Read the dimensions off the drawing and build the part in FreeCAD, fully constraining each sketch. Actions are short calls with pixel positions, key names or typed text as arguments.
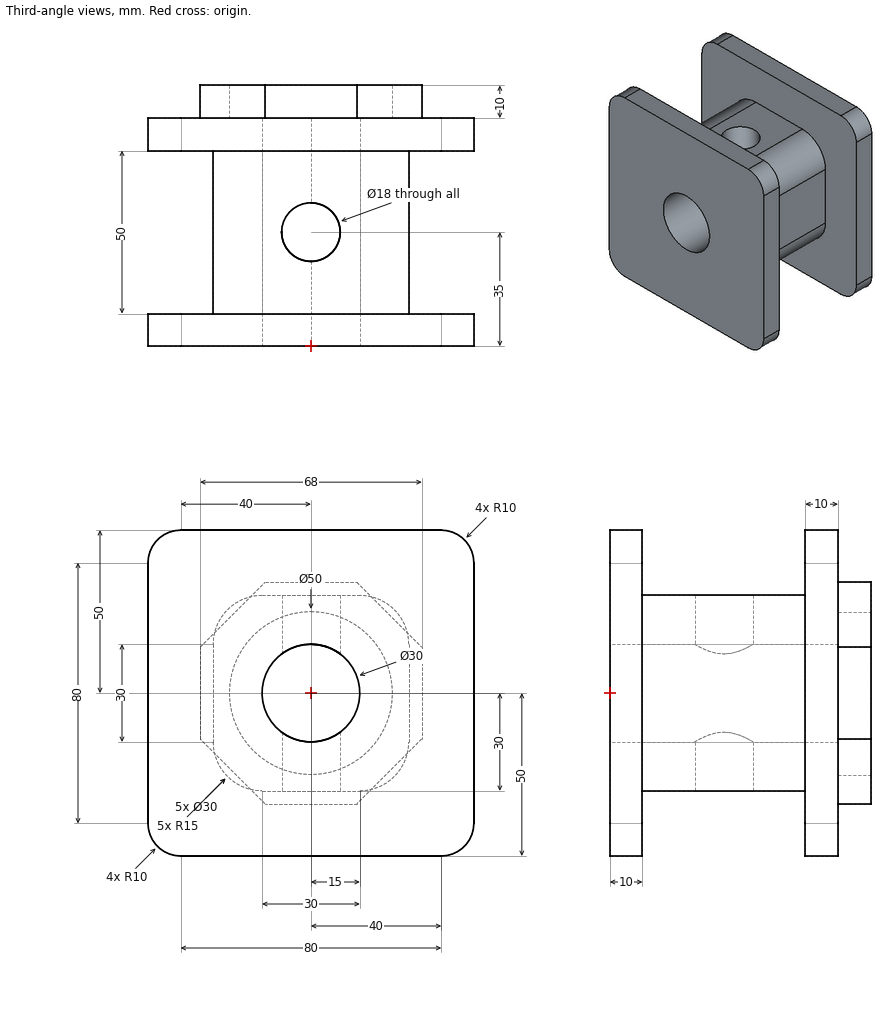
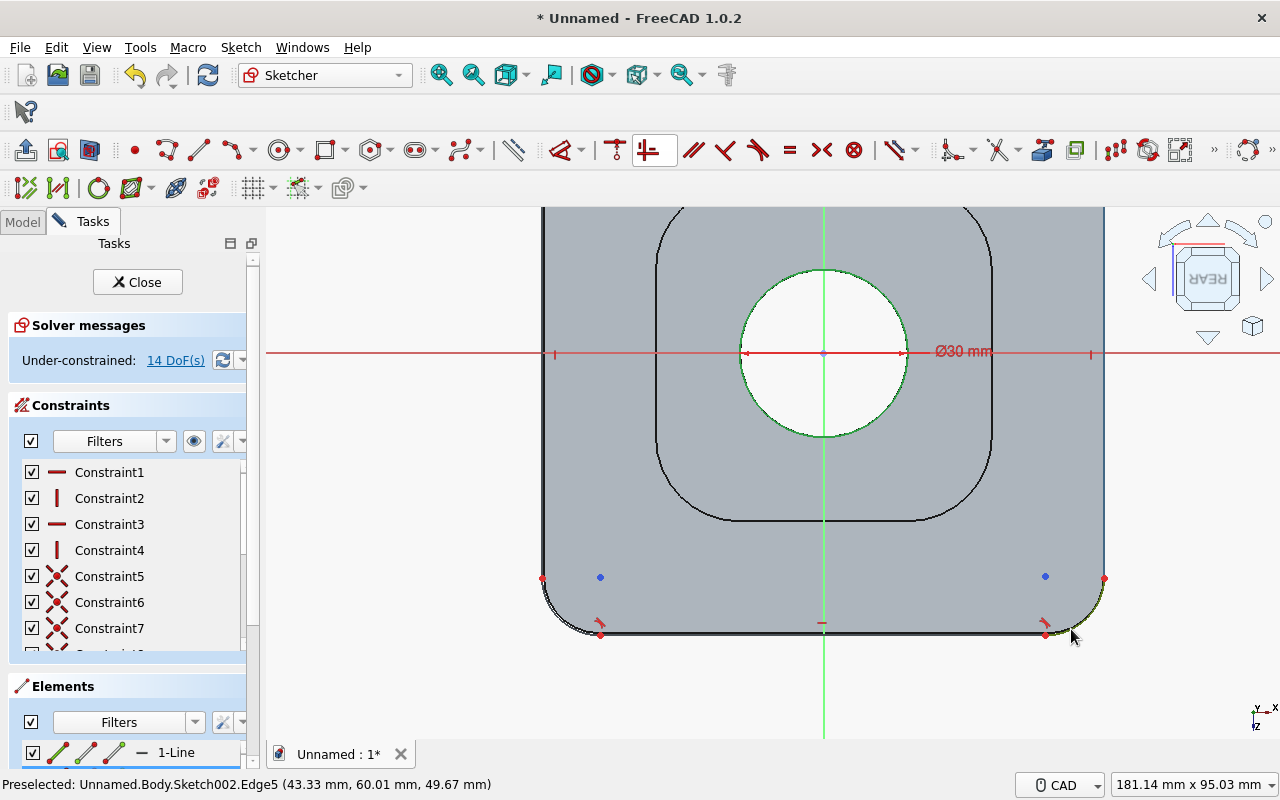
click(758, 150)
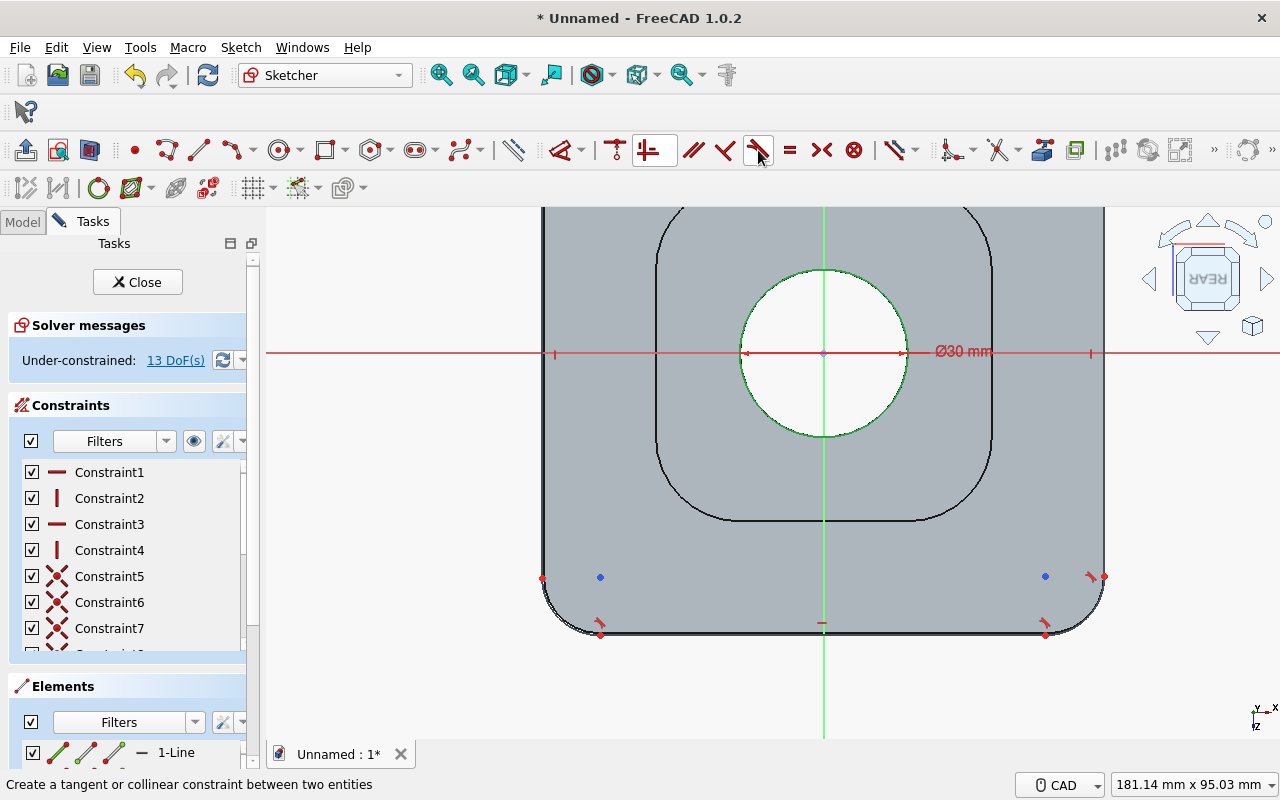
click(1104, 443)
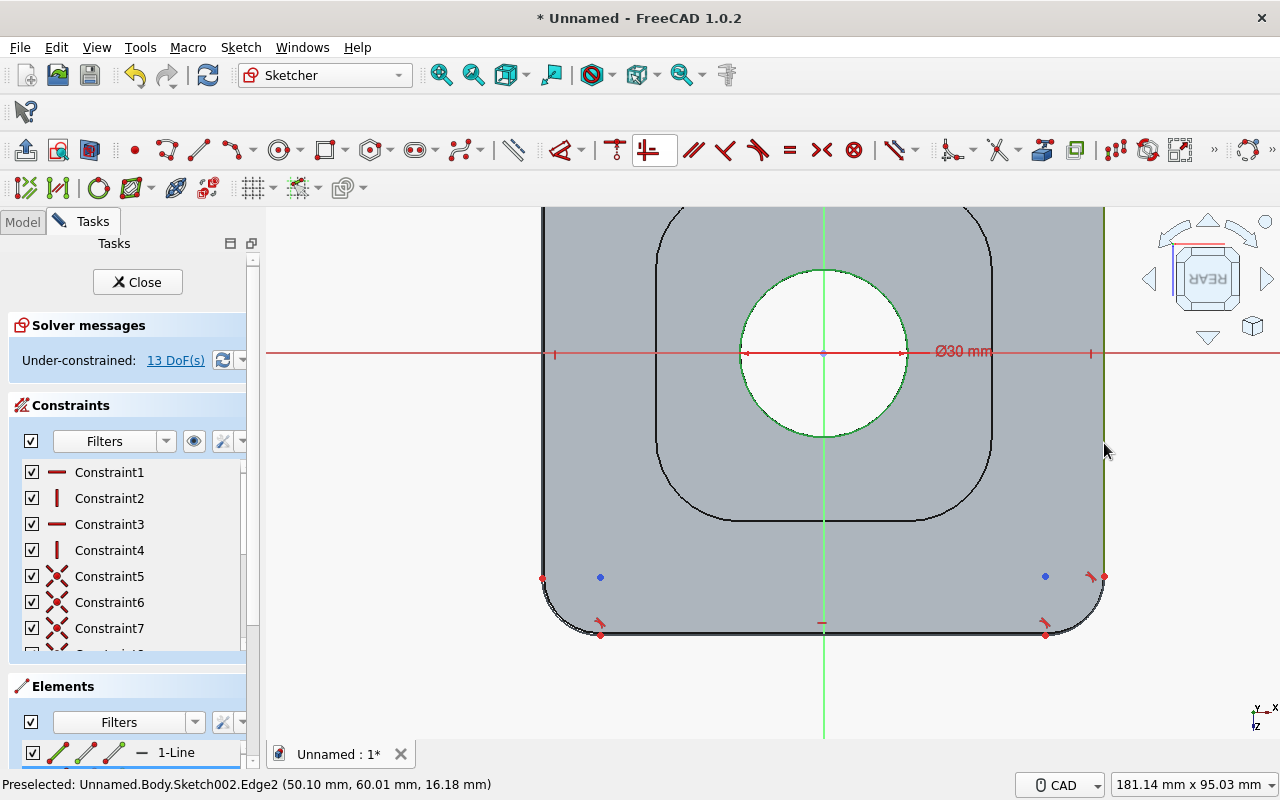
scroll(559, 618, down, 3)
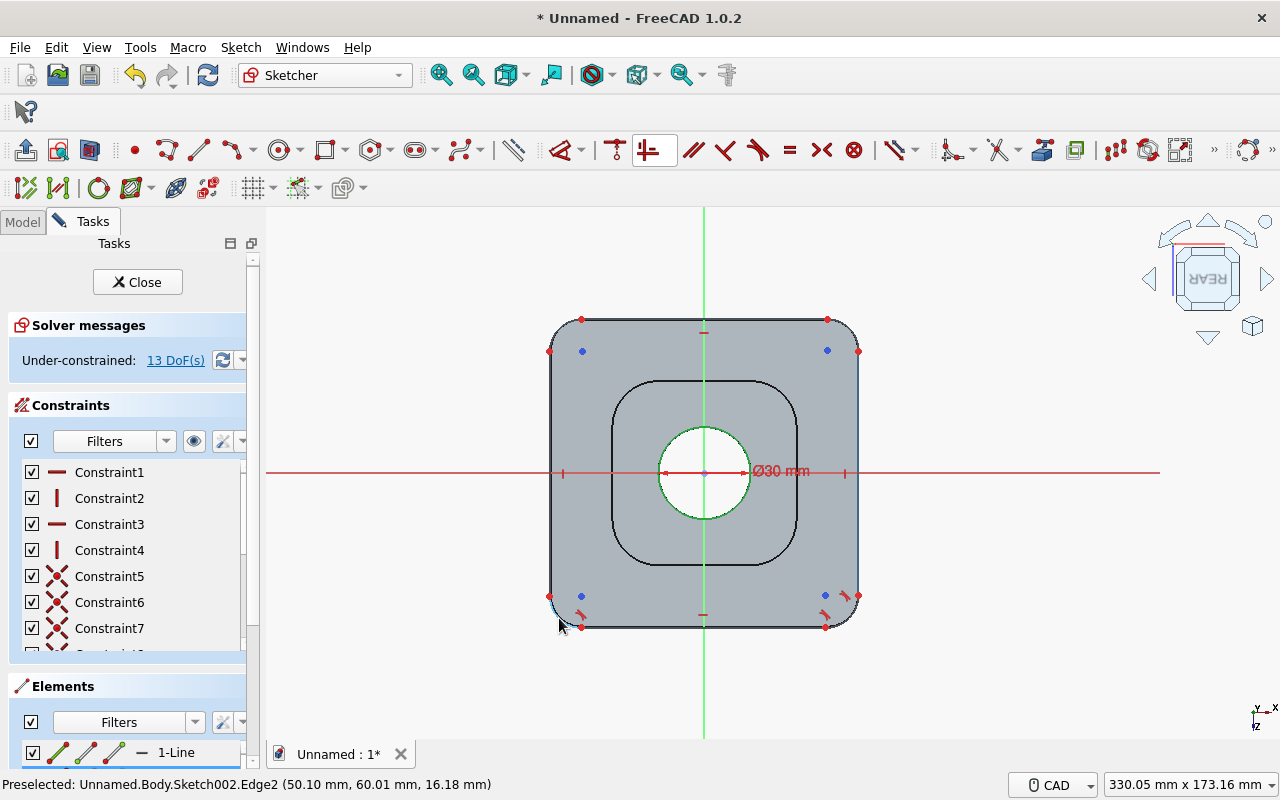
click(855, 337)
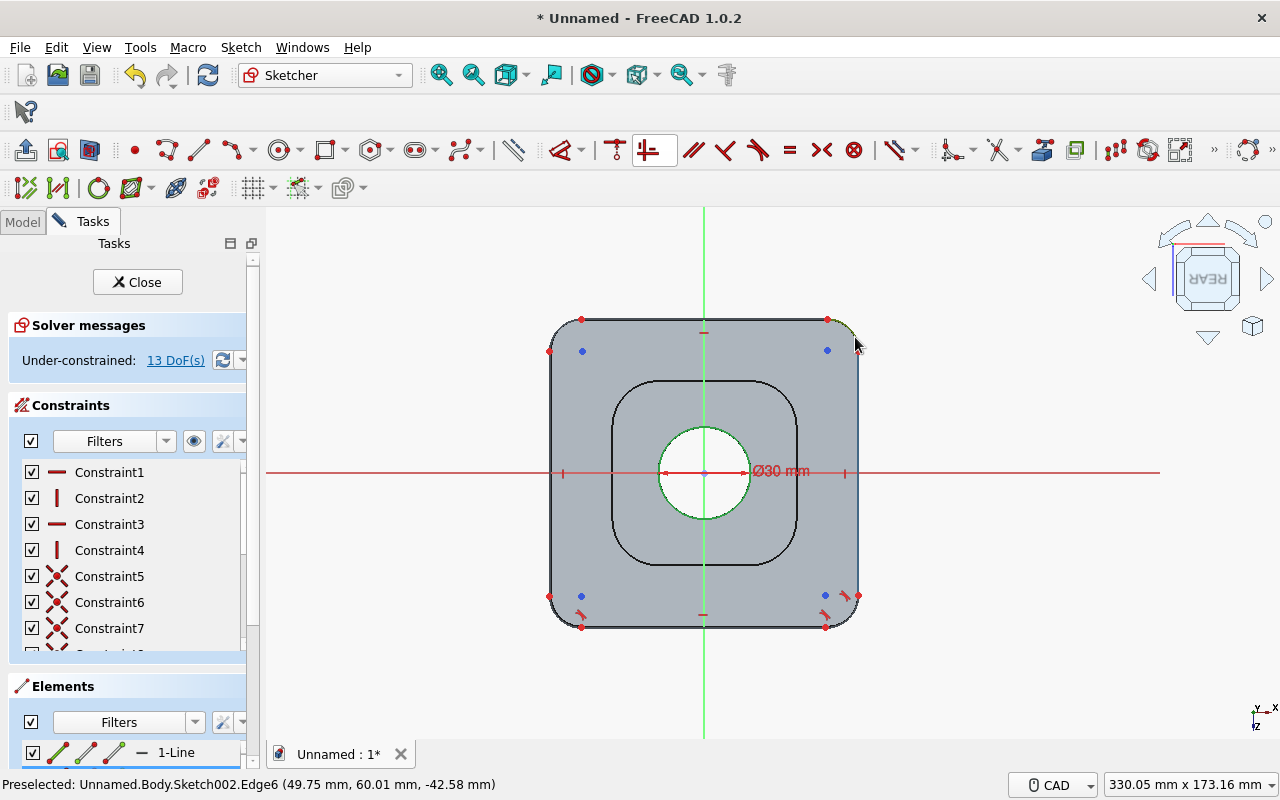
click(758, 150)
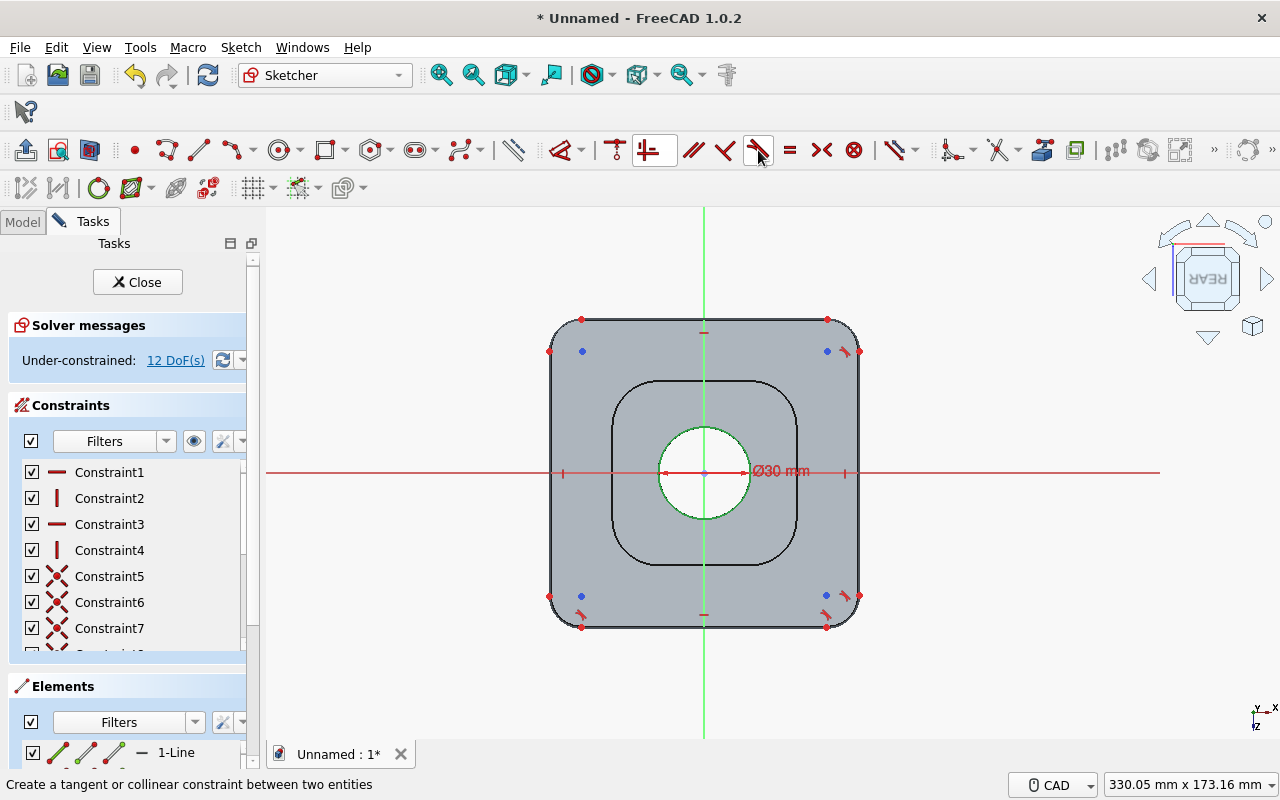
click(754, 319)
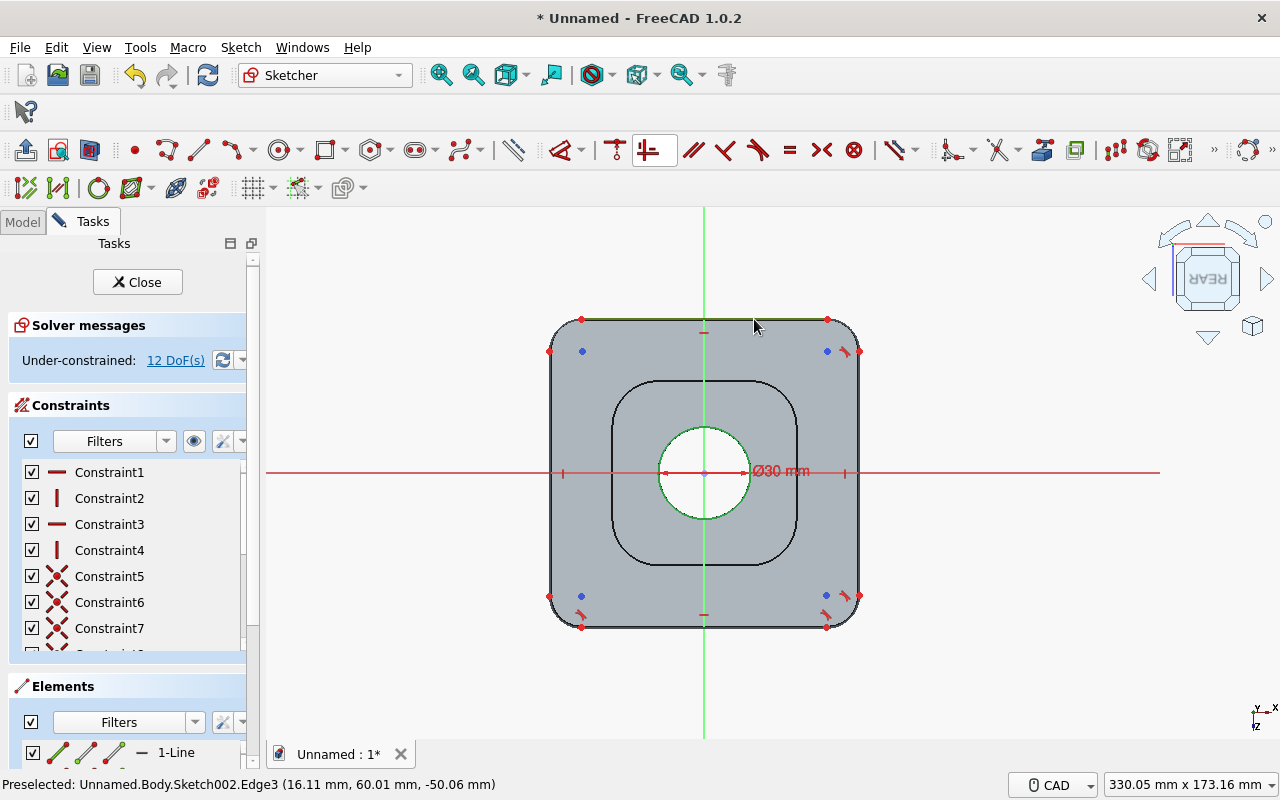
click(856, 337)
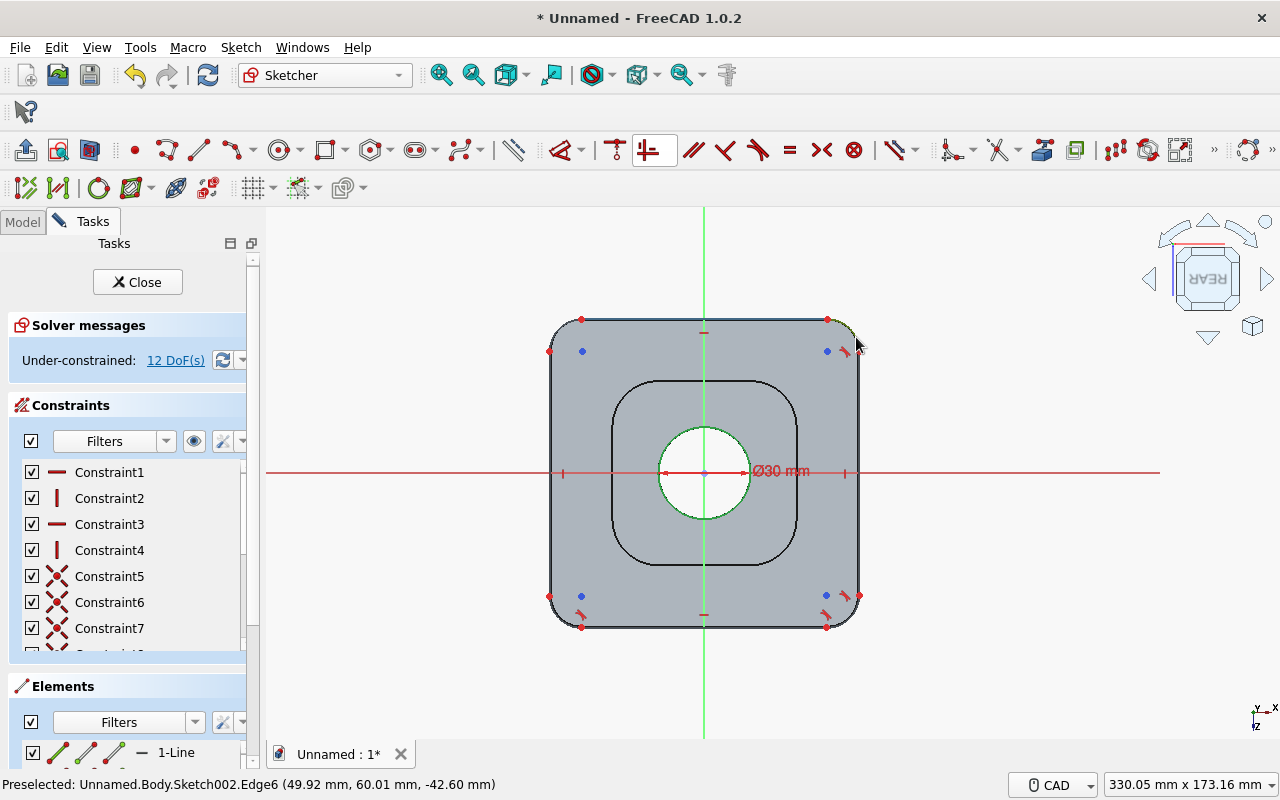
click(758, 150)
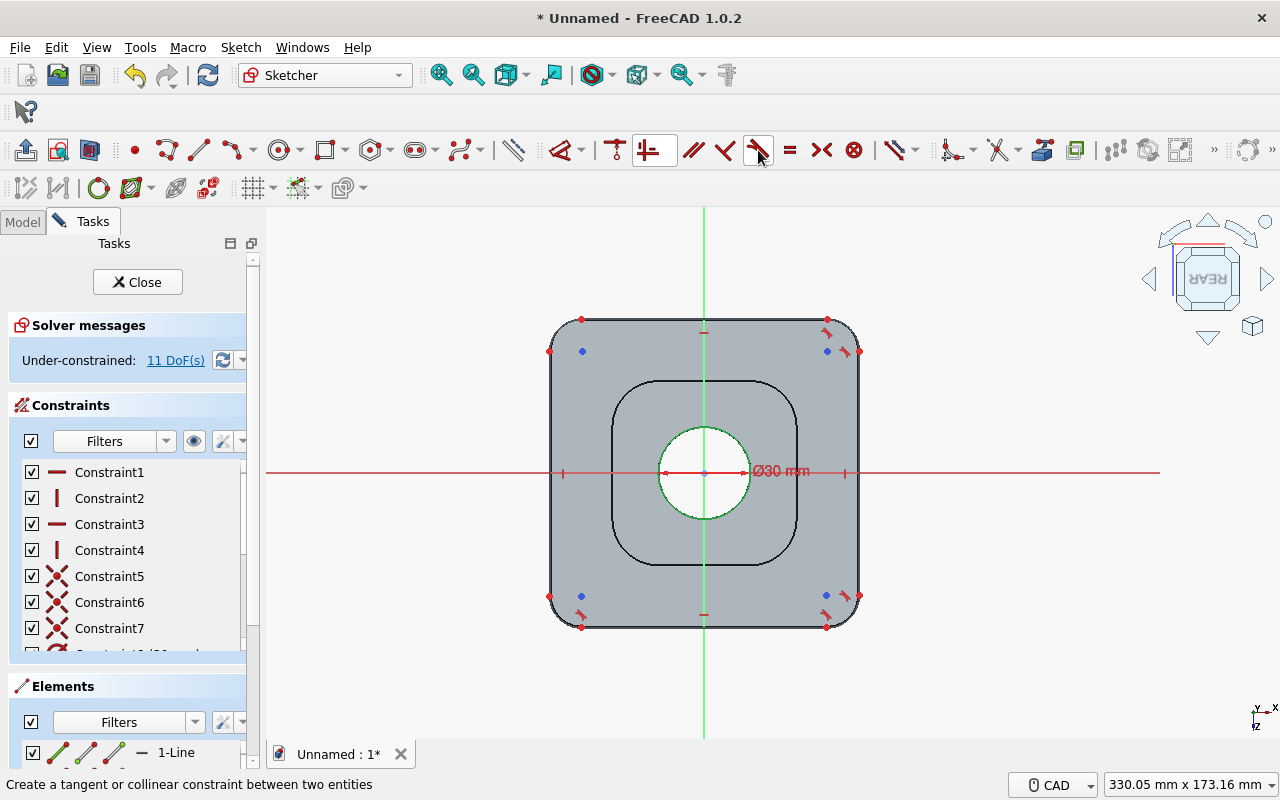
click(754, 319)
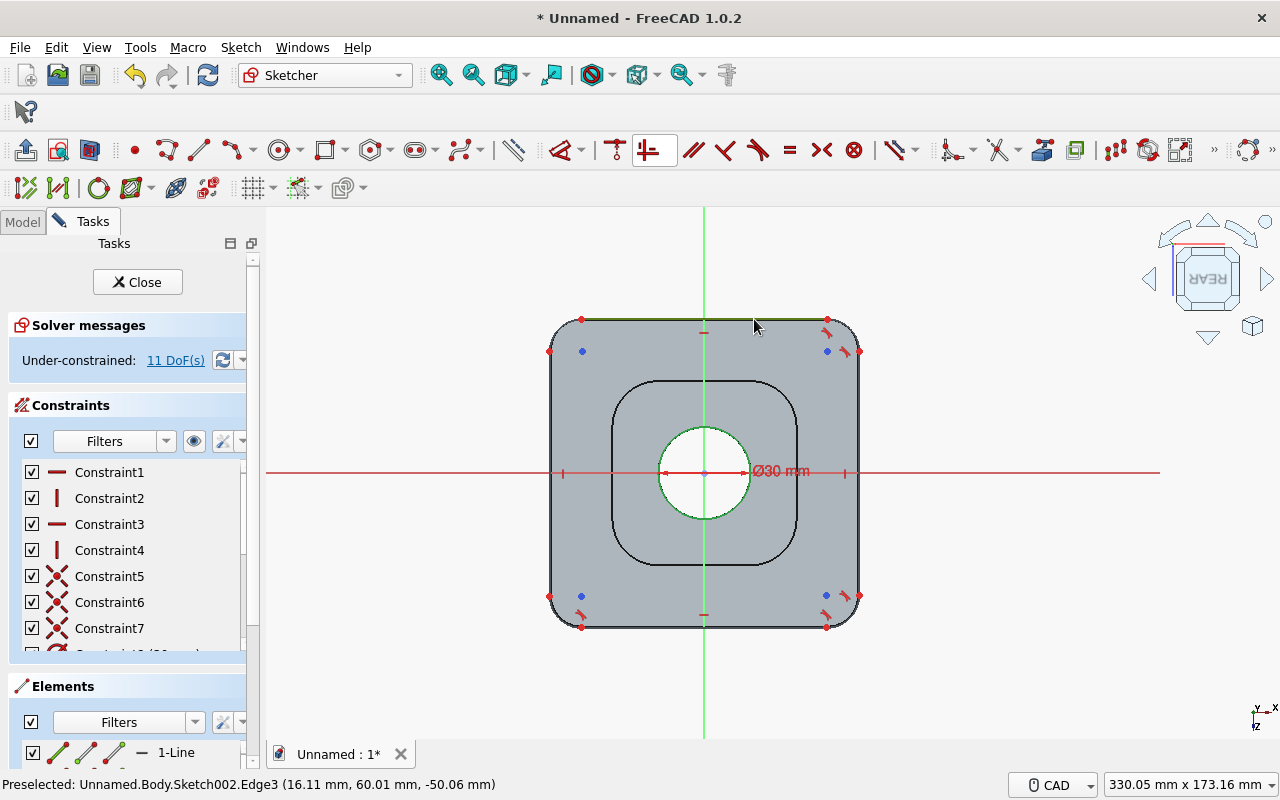
click(567, 323)